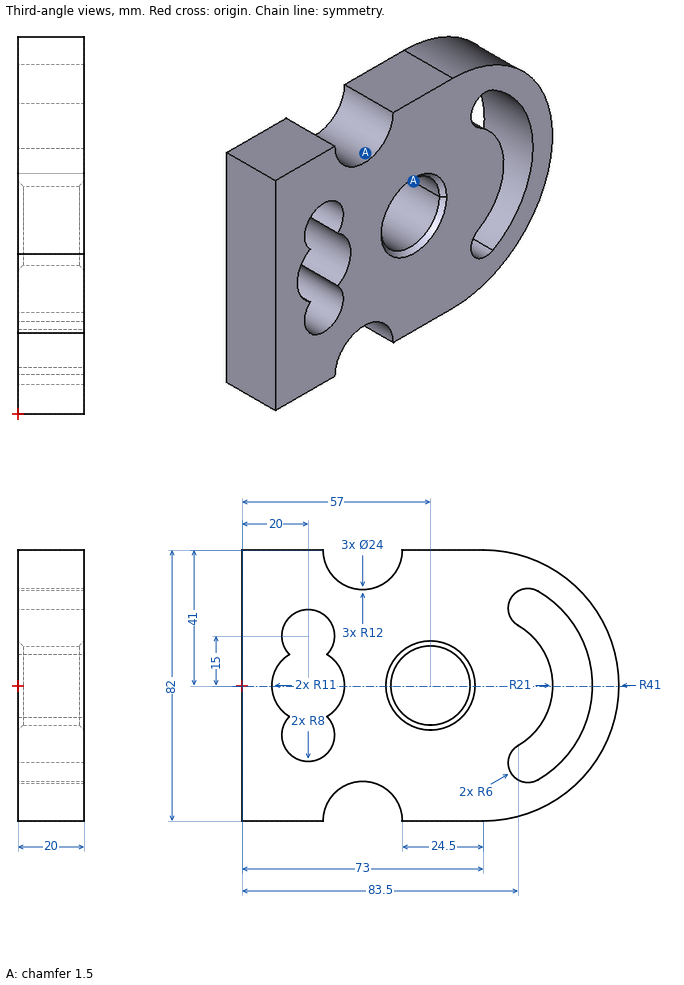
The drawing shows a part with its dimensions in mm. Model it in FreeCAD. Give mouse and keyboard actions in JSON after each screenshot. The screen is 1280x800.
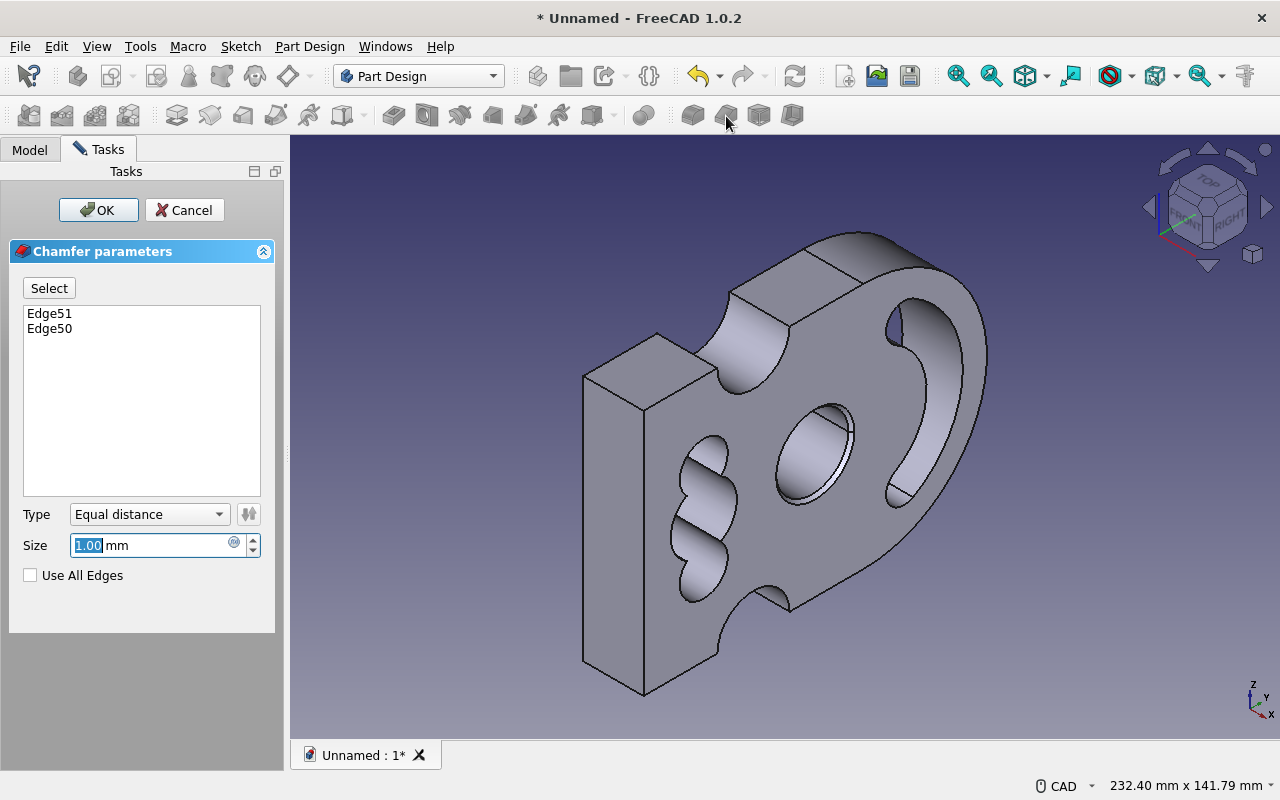
{"action": "type", "text": "1.5"}
{"action": "key", "text": "Tab"}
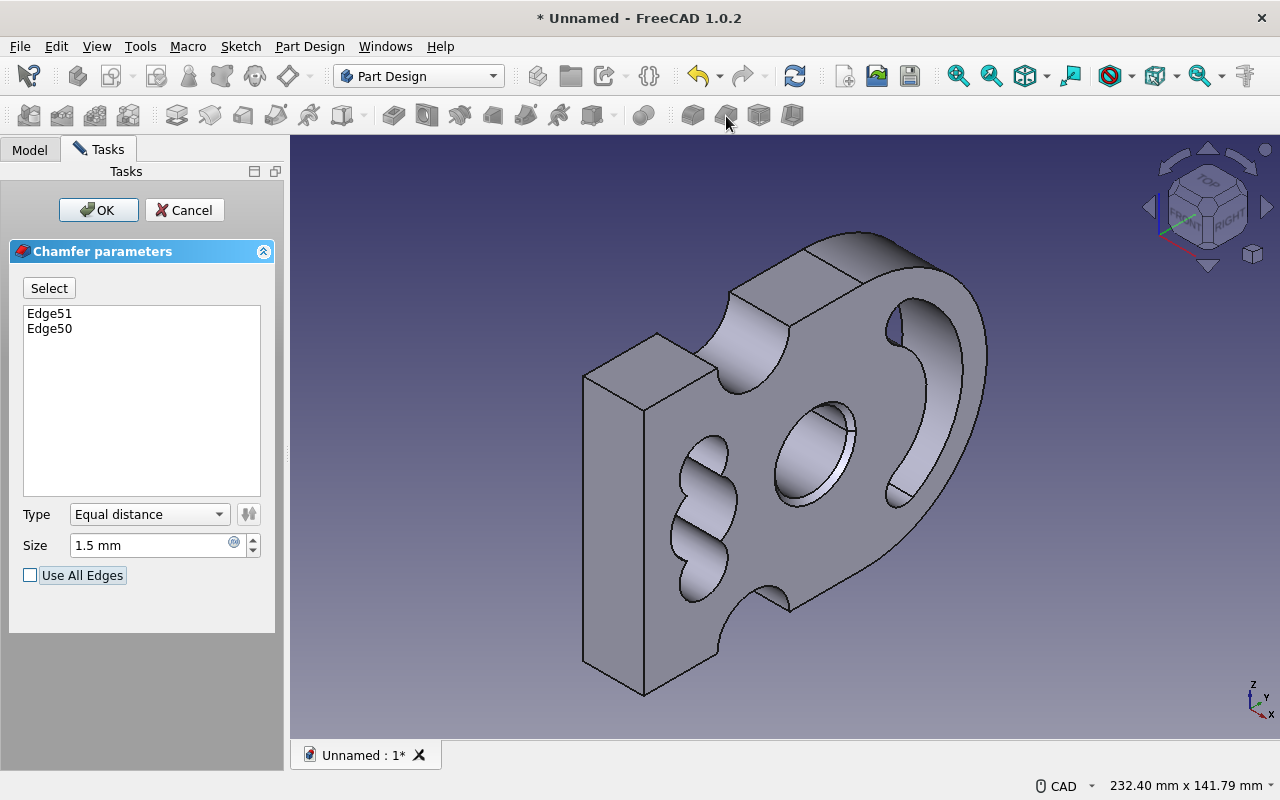
{"action": "left_click", "coordinate": [99, 210]}